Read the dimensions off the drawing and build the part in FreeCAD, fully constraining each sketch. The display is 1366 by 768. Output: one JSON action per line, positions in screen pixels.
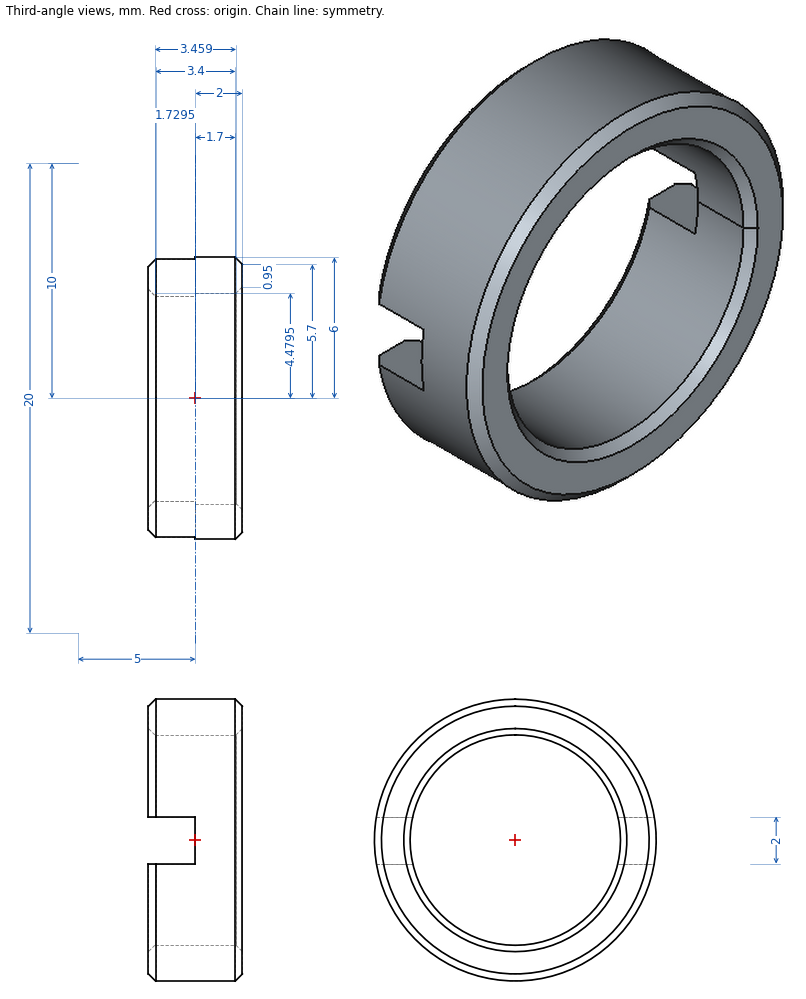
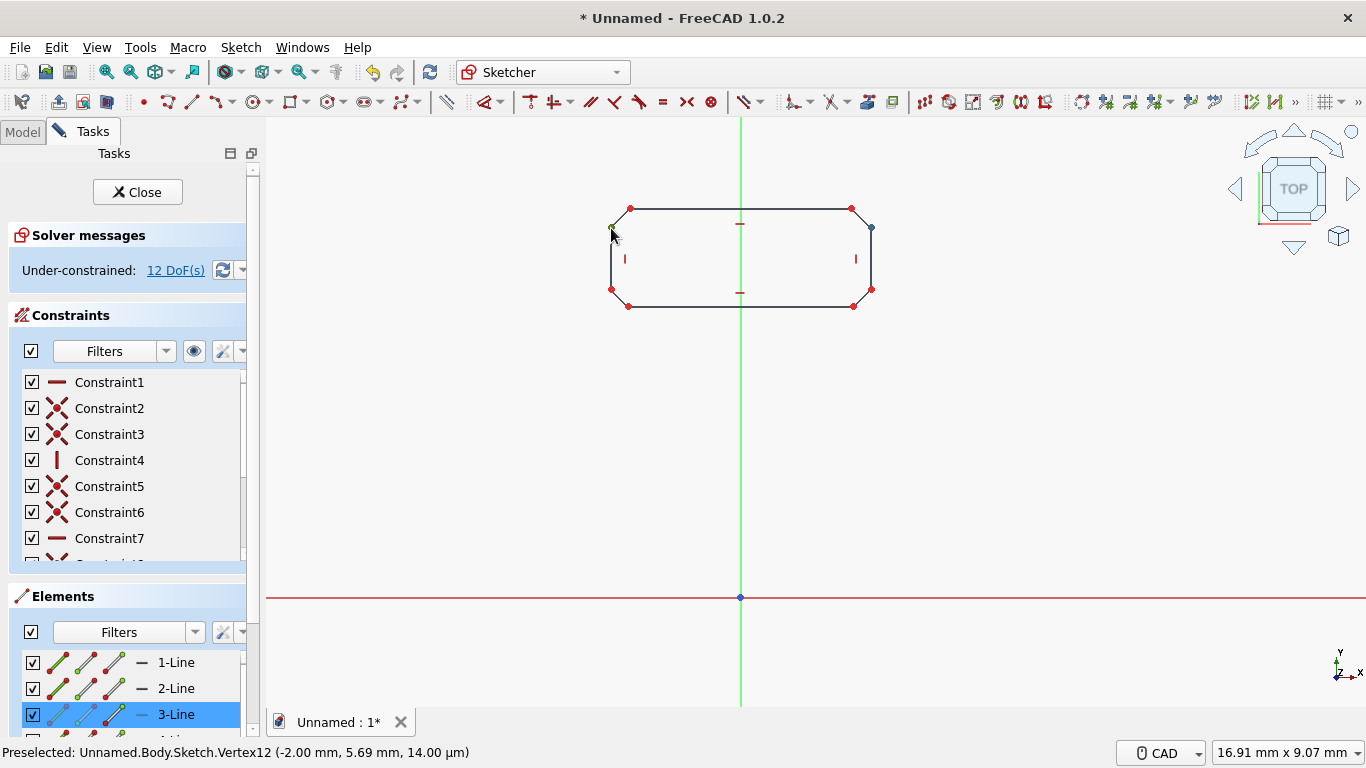
{"action": "left_click", "coordinate": [741, 641]}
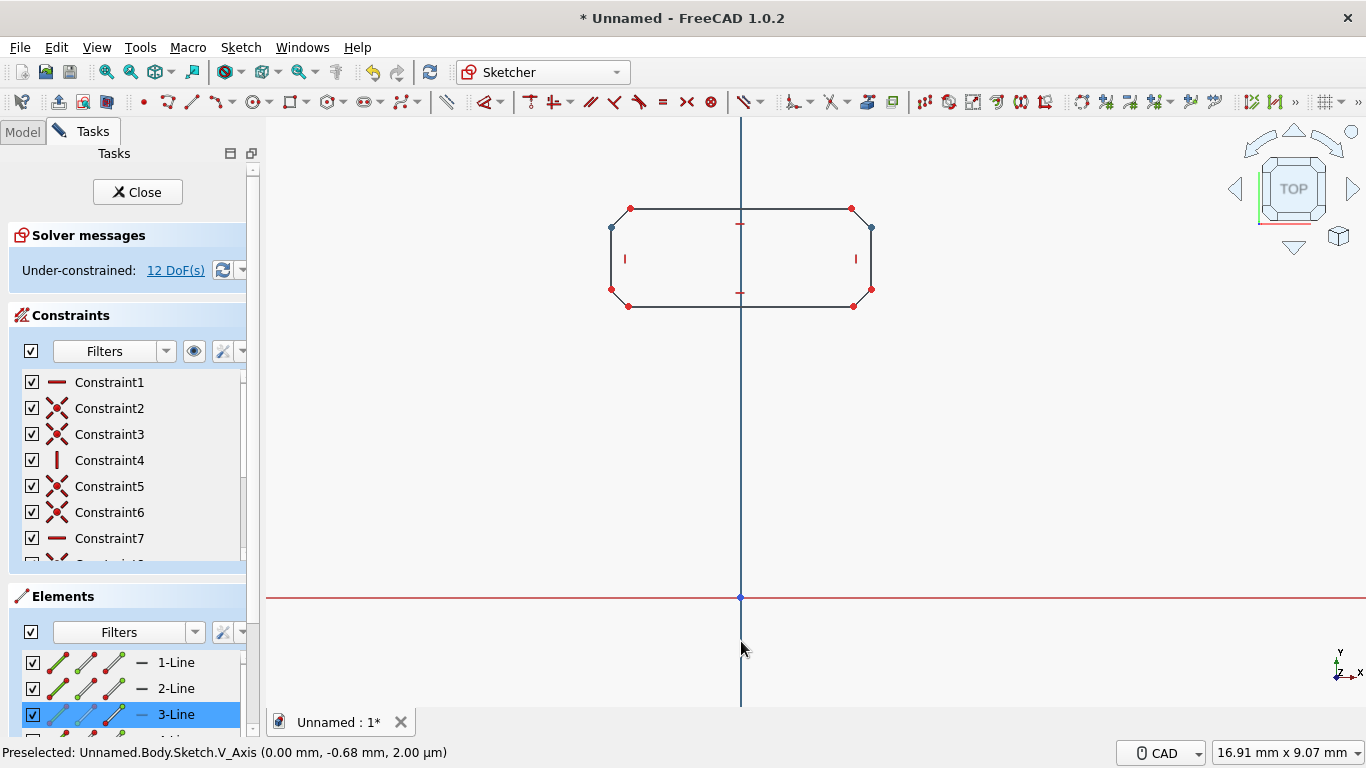
{"action": "key", "text": "s"}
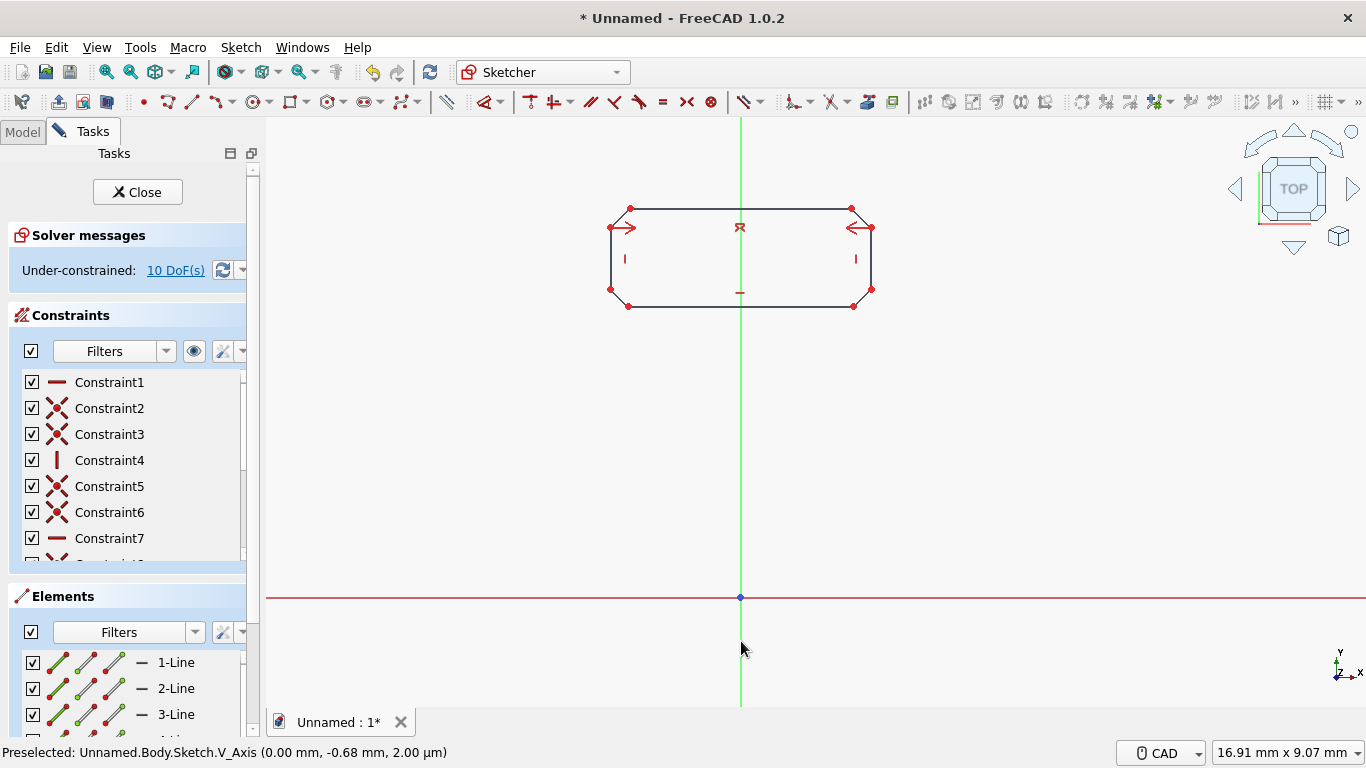
{"action": "left_click", "coordinate": [484, 102]}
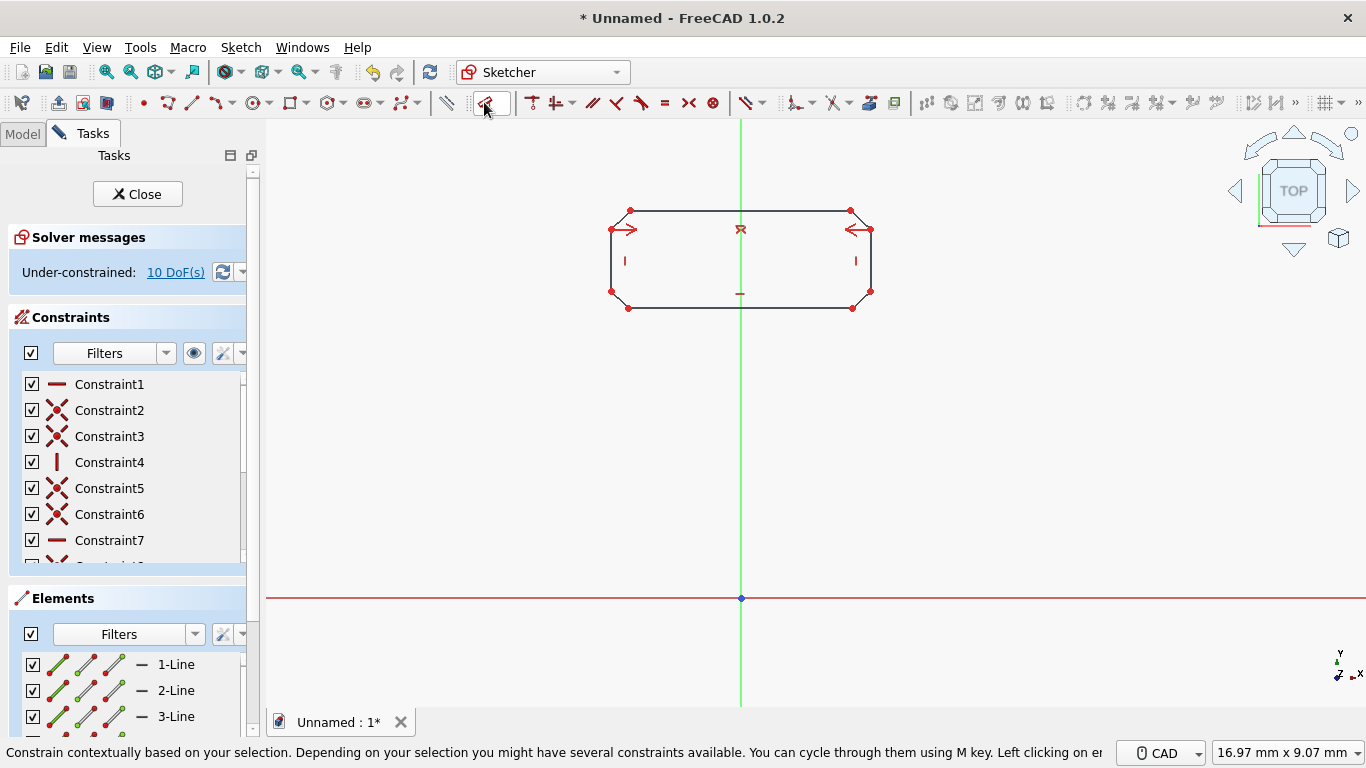
{"action": "left_click", "coordinate": [871, 291]}
{"action": "left_click", "coordinate": [806, 632]}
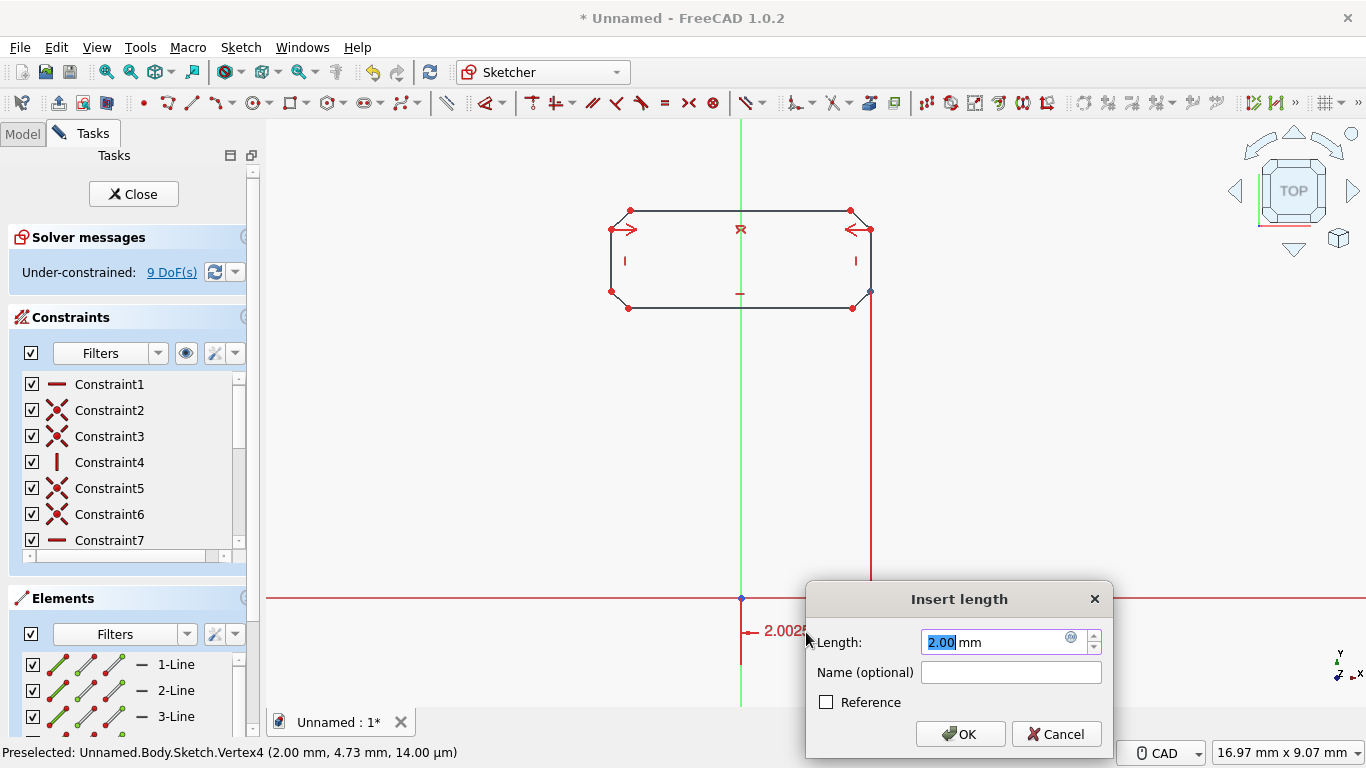
{"action": "type", "text": "2"}
{"action": "key", "text": "Return"}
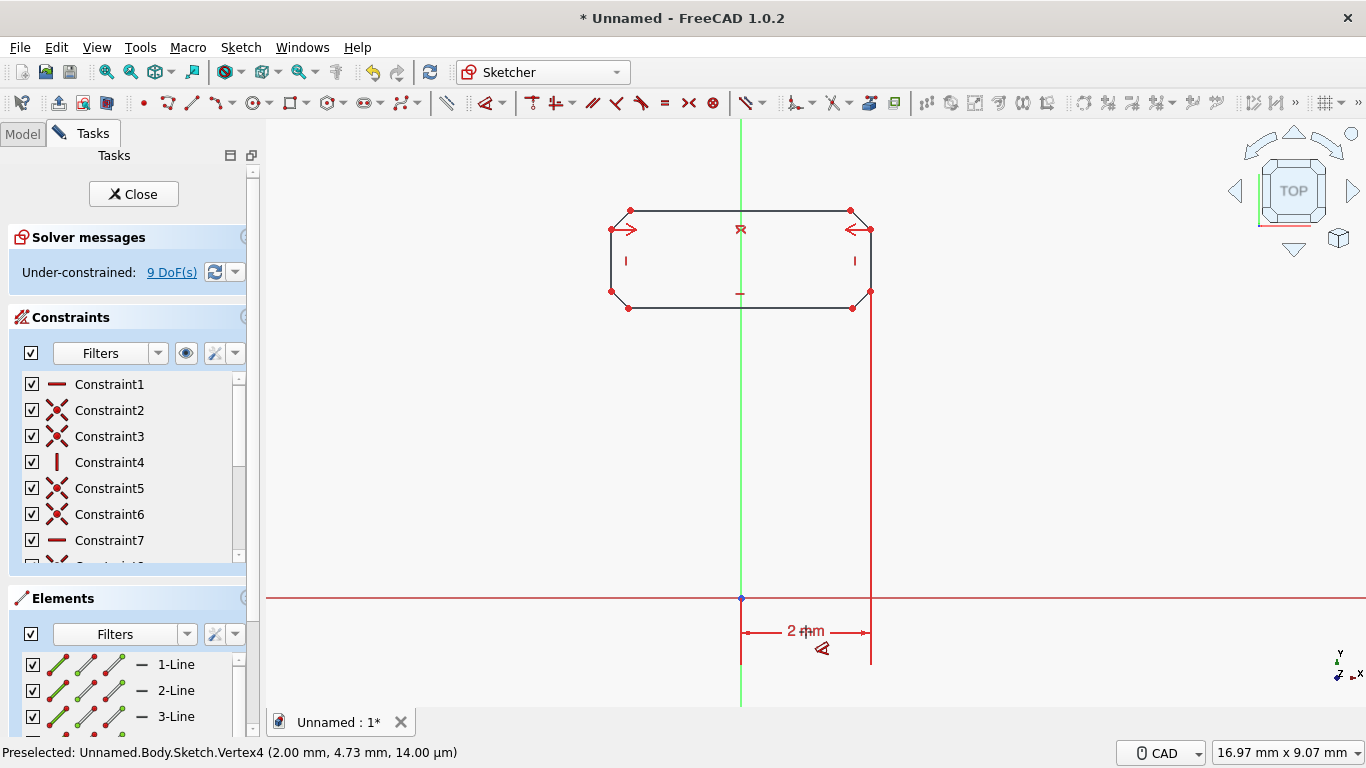
{"action": "left_click", "coordinate": [851, 211]}
{"action": "left_click", "coordinate": [885, 404]}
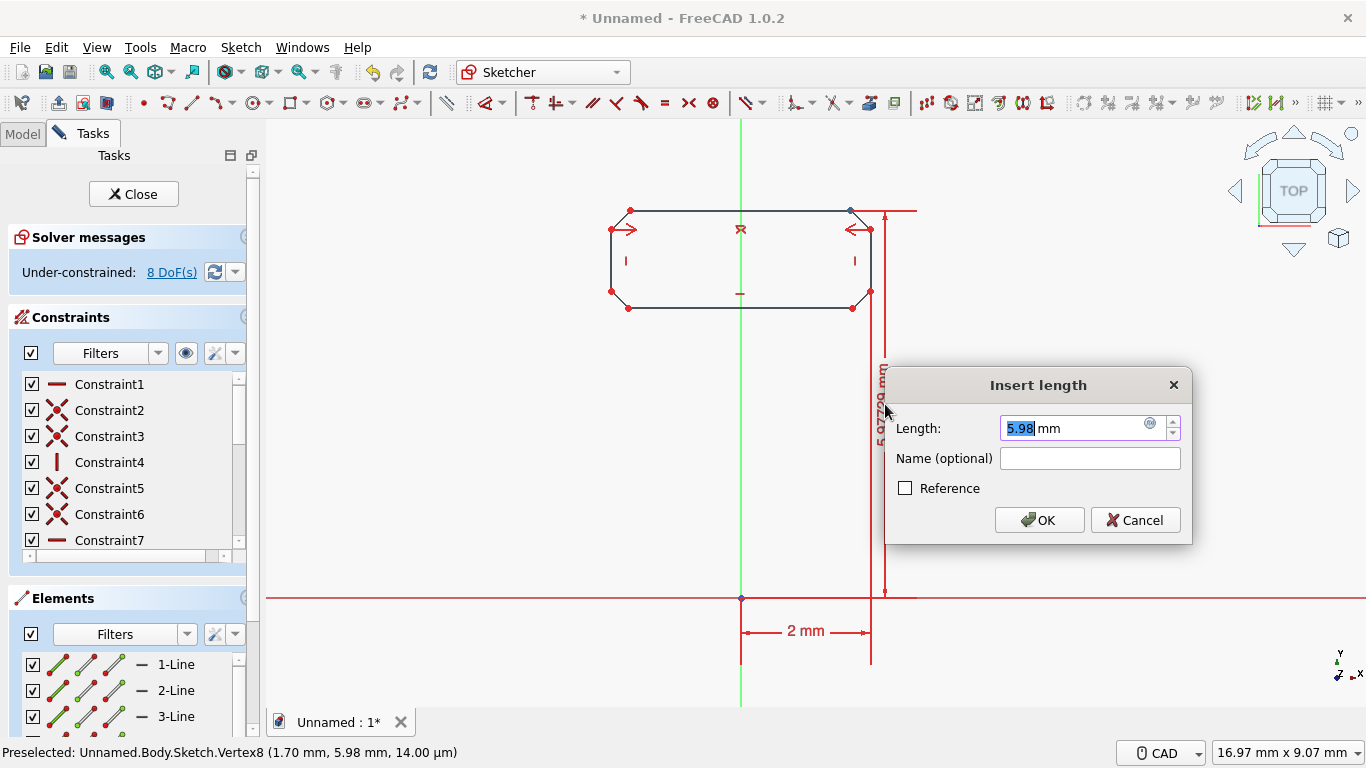
{"action": "type", "text": "6"}
{"action": "key", "text": "Return"}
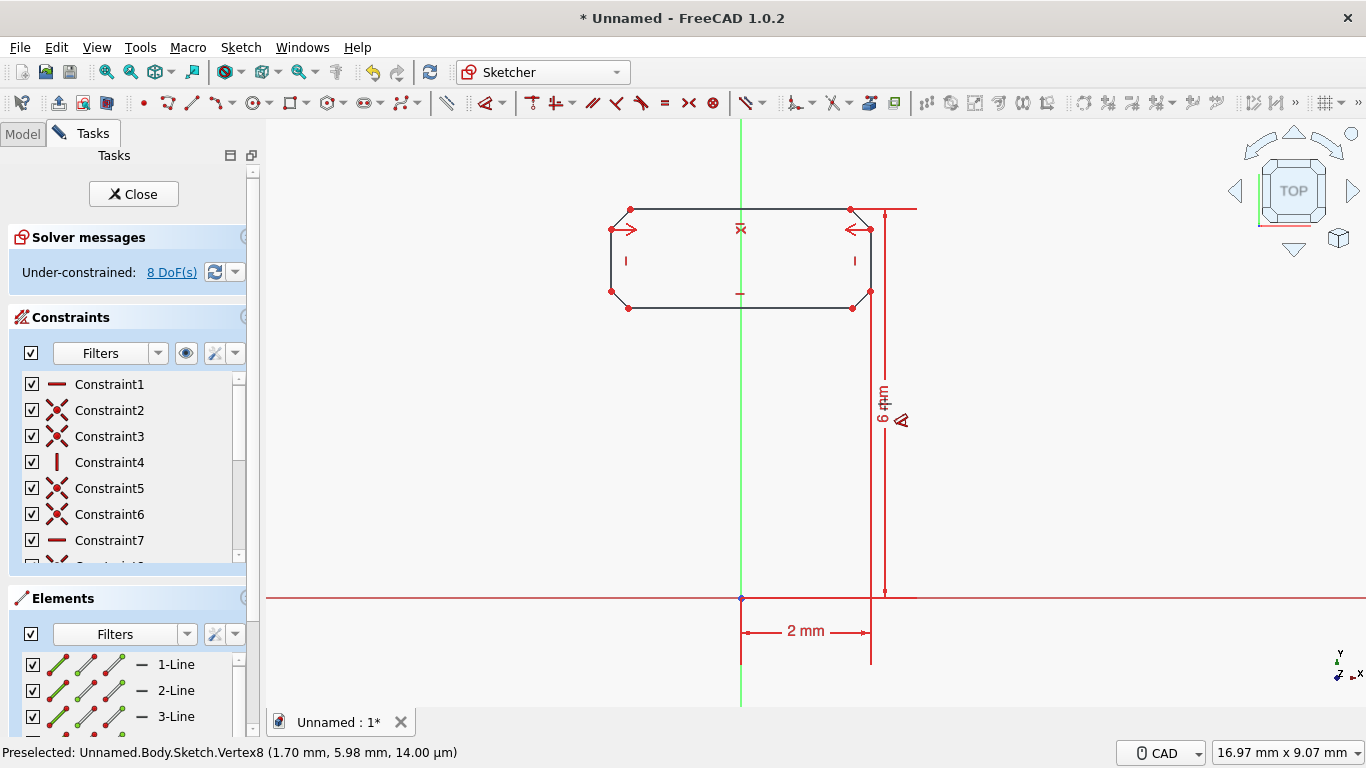
{"action": "left_click", "coordinate": [785, 209]}
{"action": "left_click", "coordinate": [690, 175]}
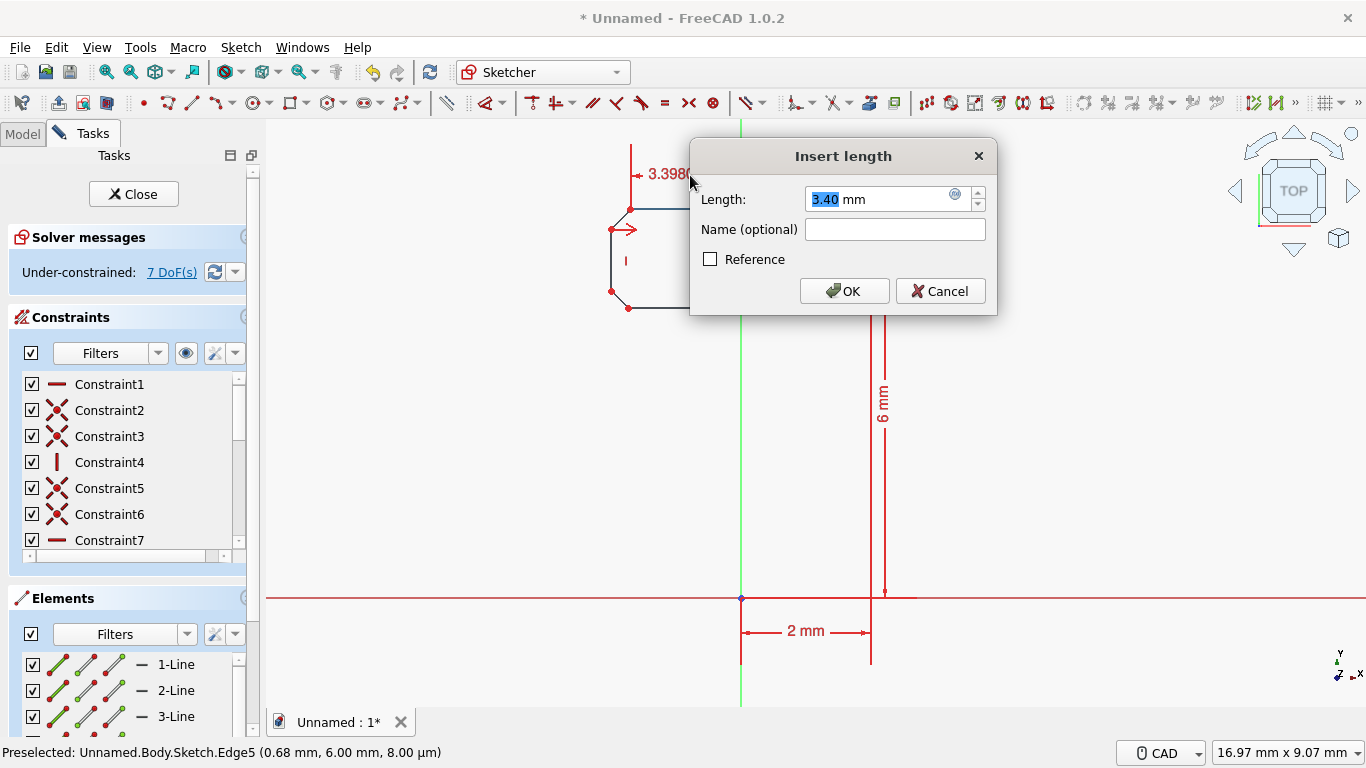
{"action": "type", "text": "3.4"}
{"action": "key", "text": "Return"}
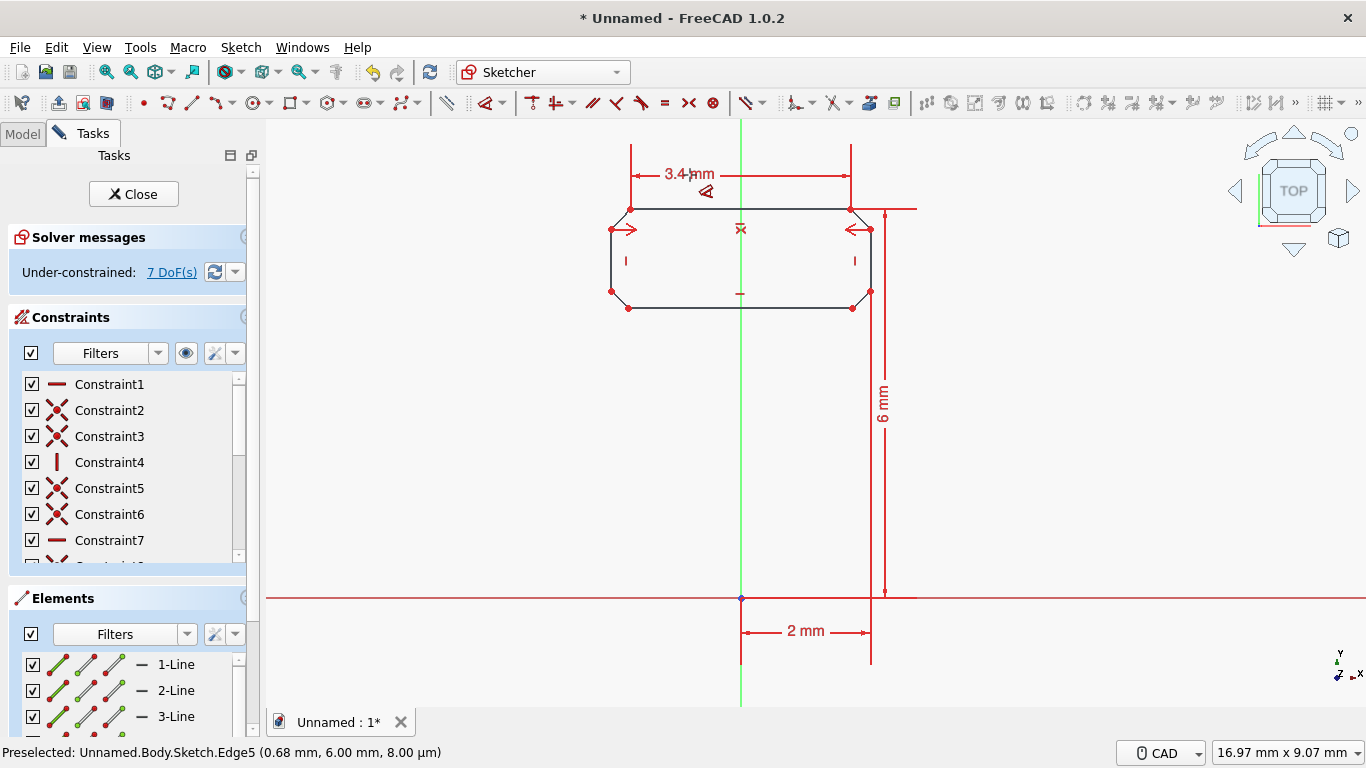
{"action": "left_click", "coordinate": [871, 273]}
{"action": "left_click", "coordinate": [905, 261]}